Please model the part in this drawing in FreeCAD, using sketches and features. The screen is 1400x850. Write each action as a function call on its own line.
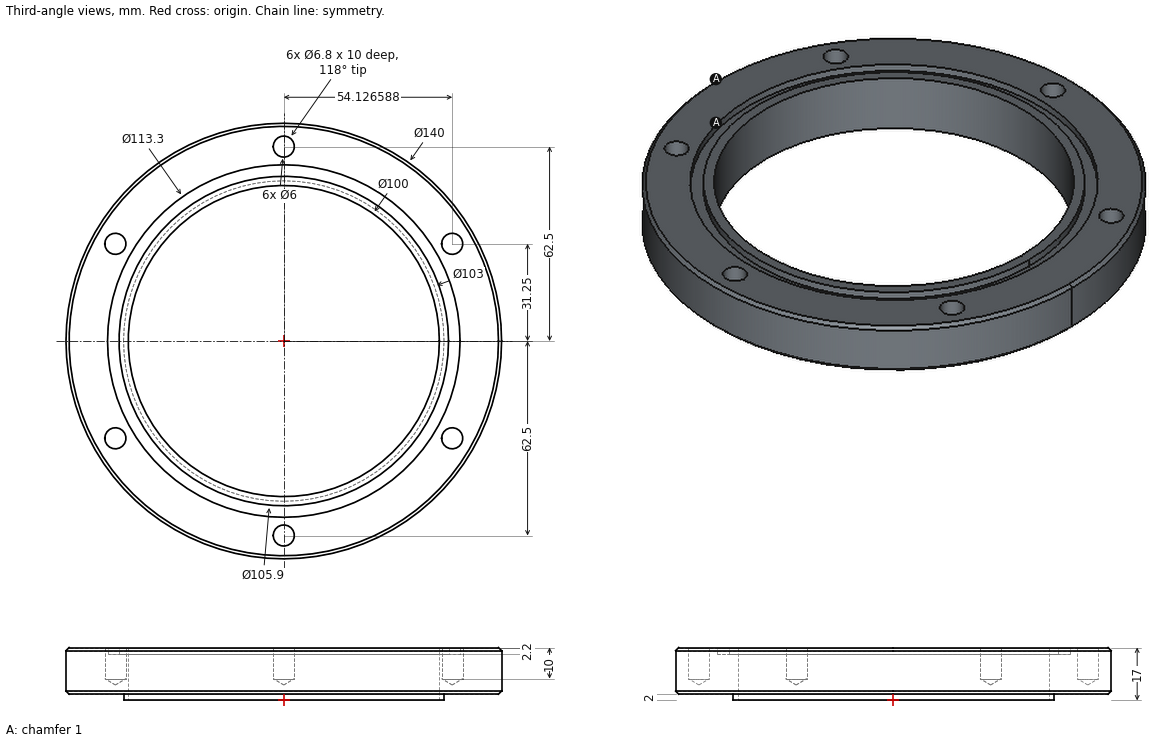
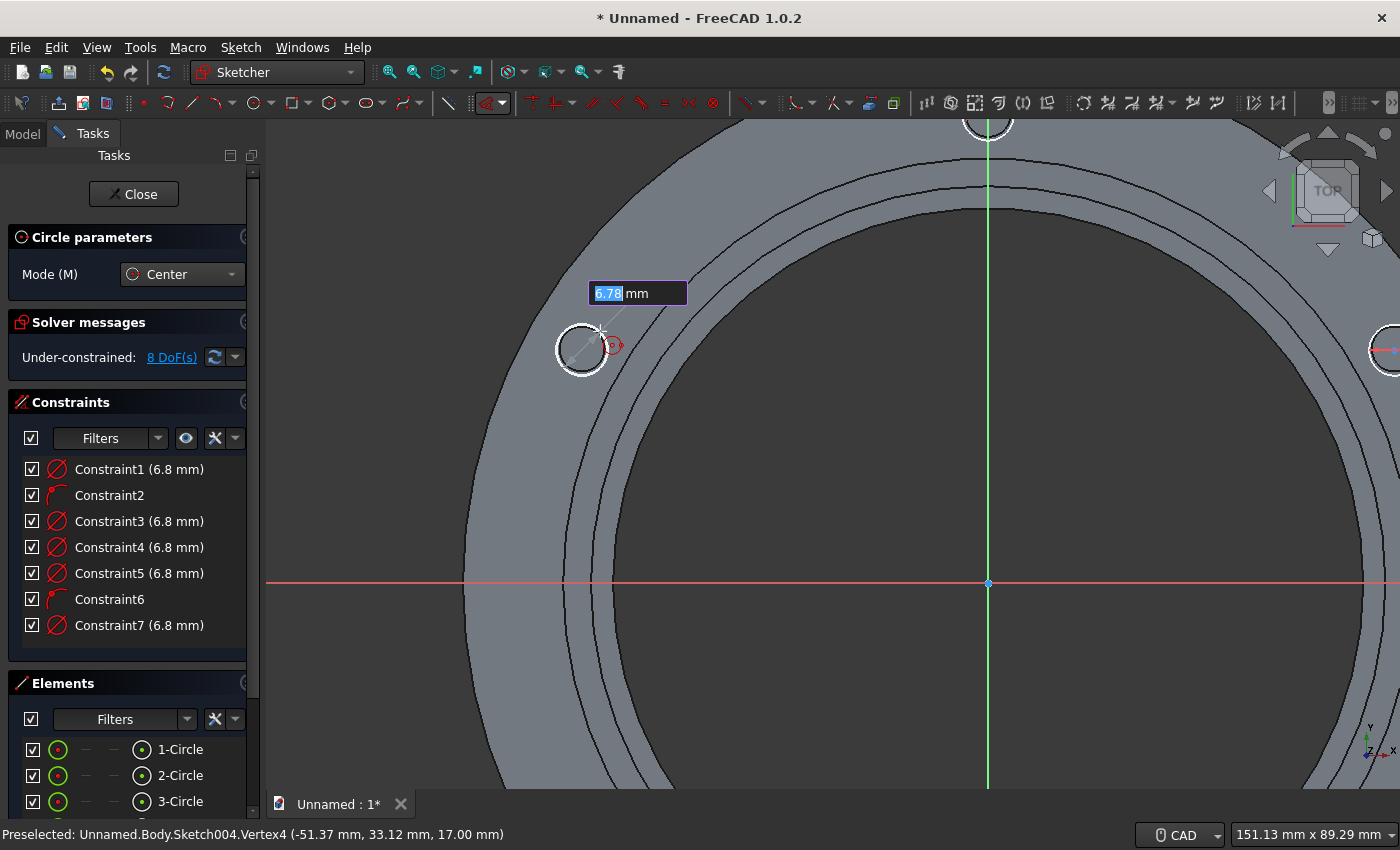
text(6.8)
key(Return)
key(Escape)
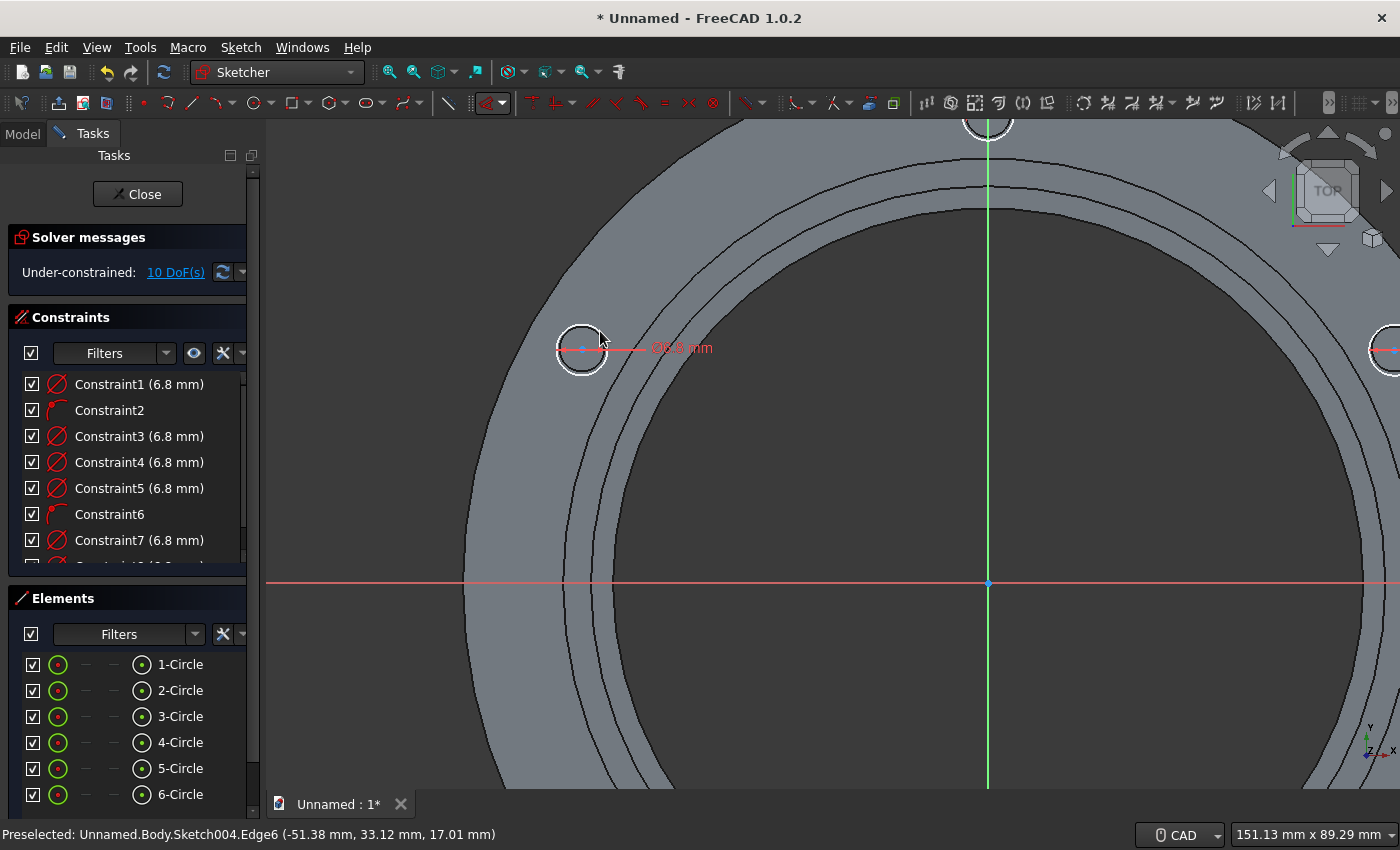
scroll(582, 348, down, 4)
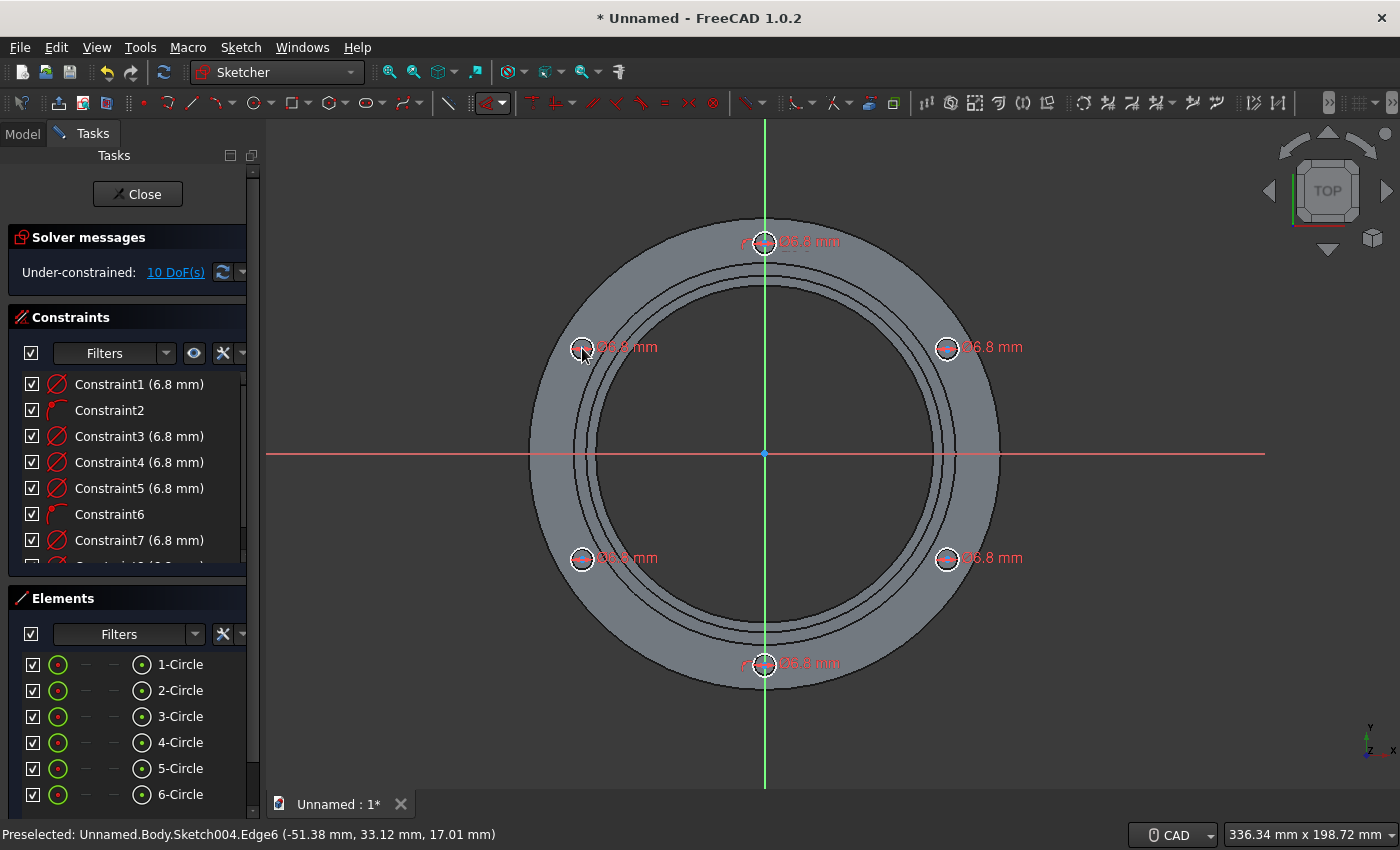
click(947, 349)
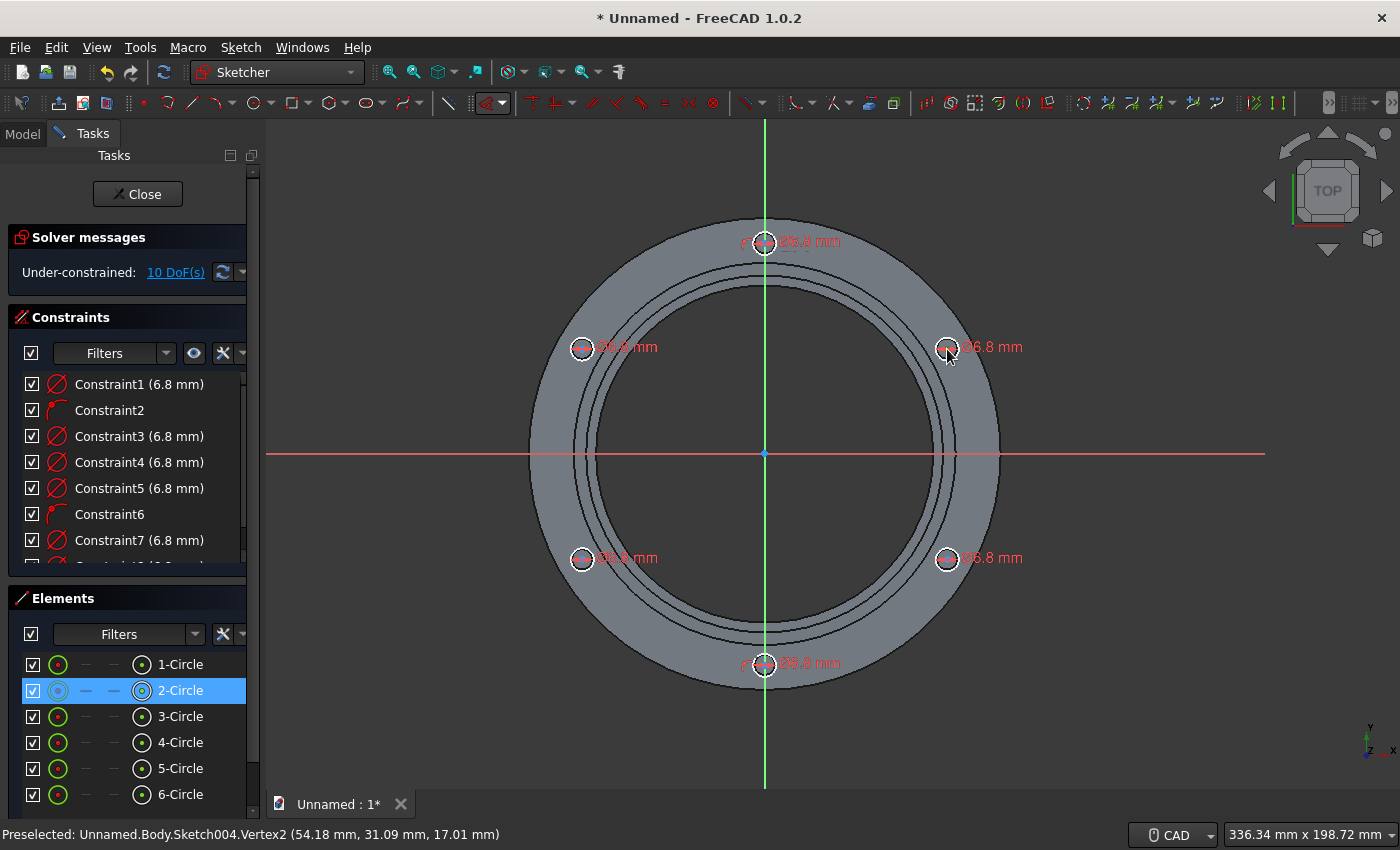
click(947, 560)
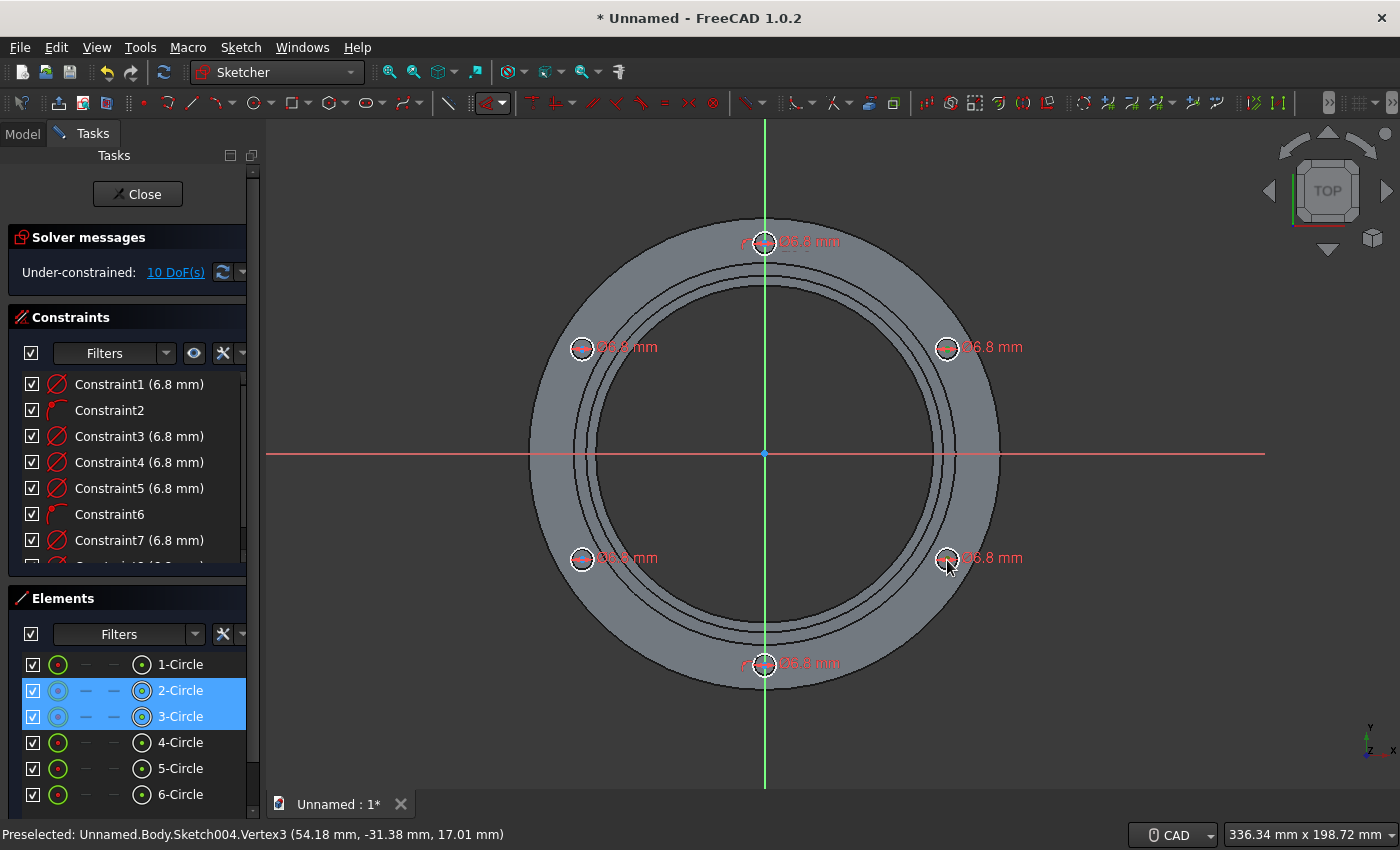
click(361, 454)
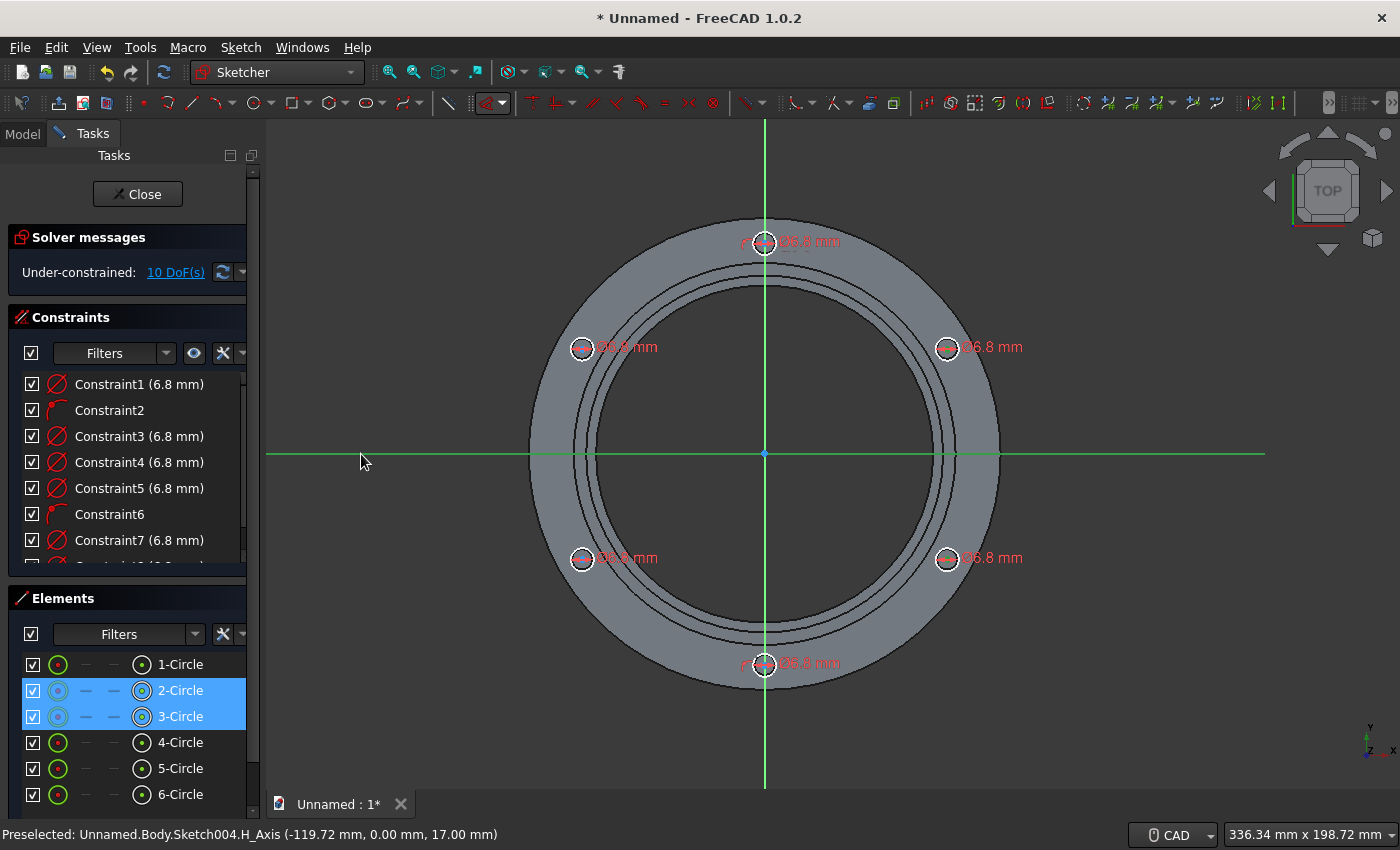
click(690, 104)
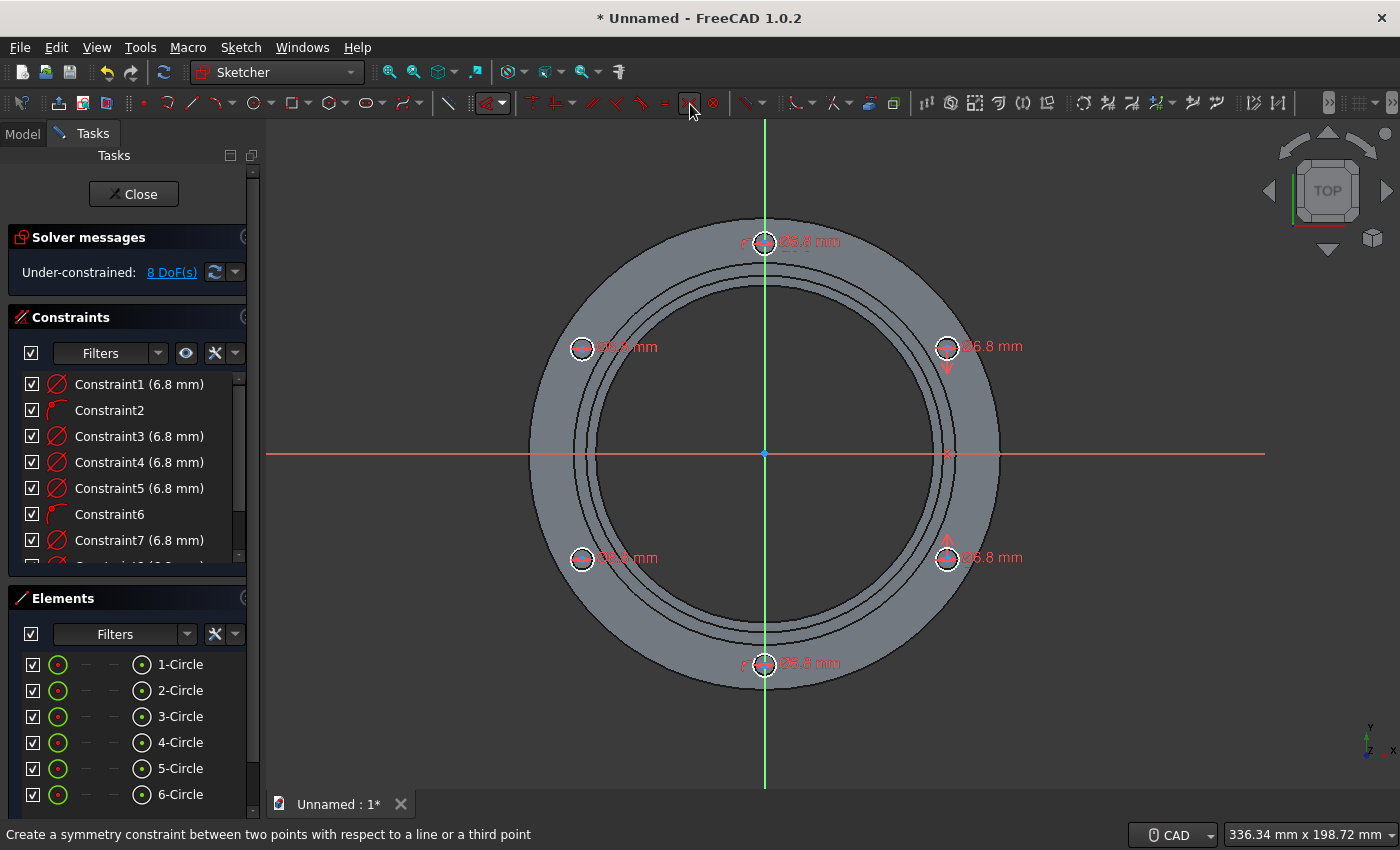
click(947, 560)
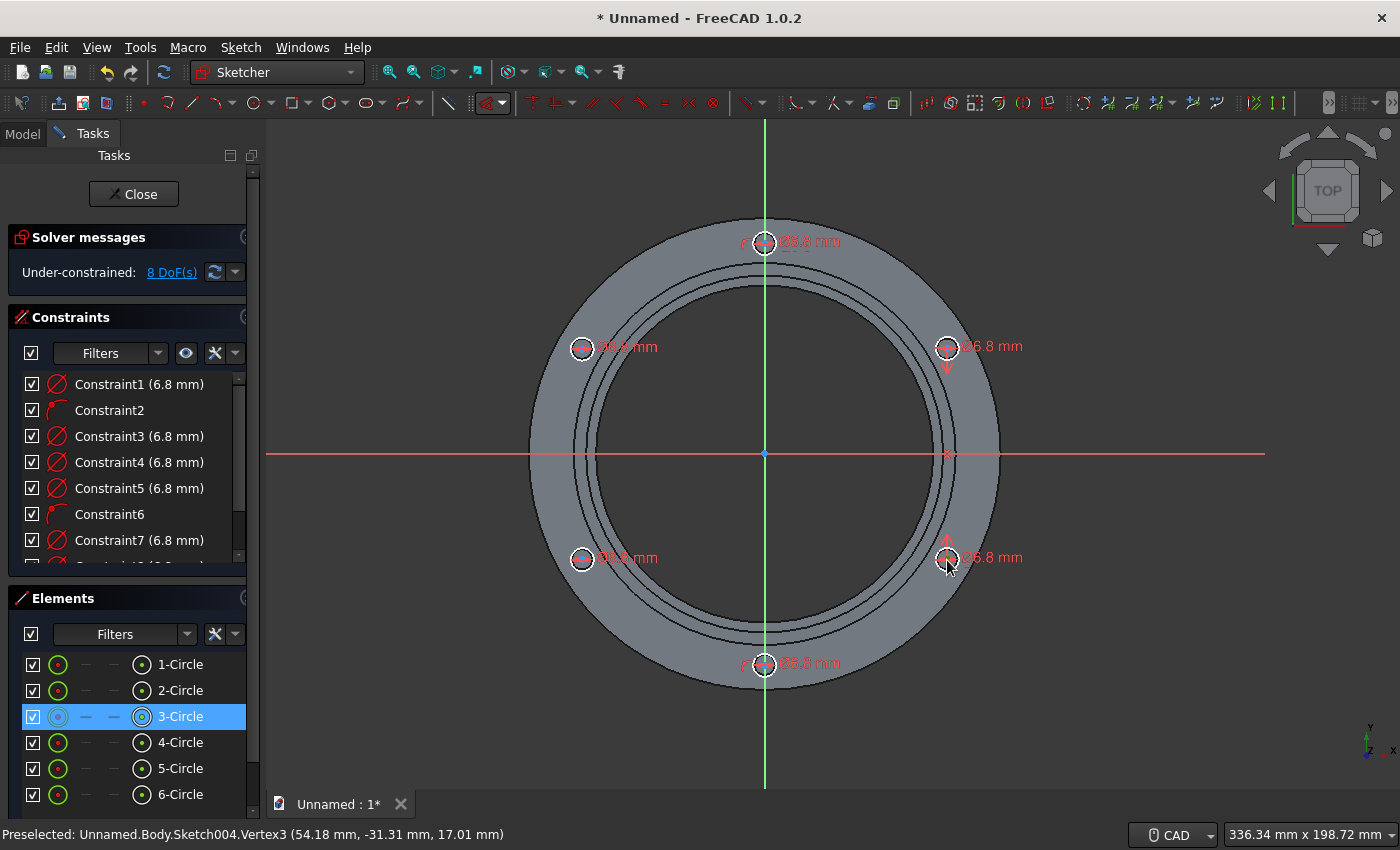
click(582, 560)